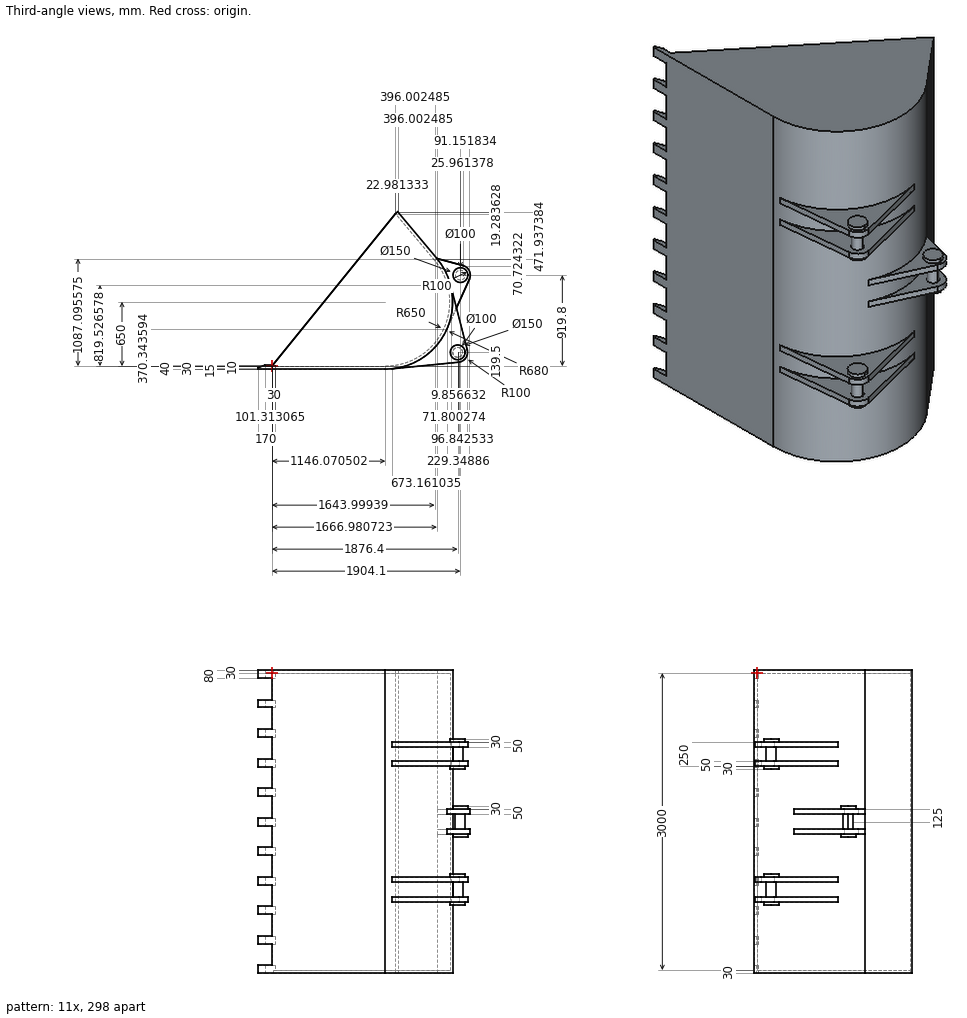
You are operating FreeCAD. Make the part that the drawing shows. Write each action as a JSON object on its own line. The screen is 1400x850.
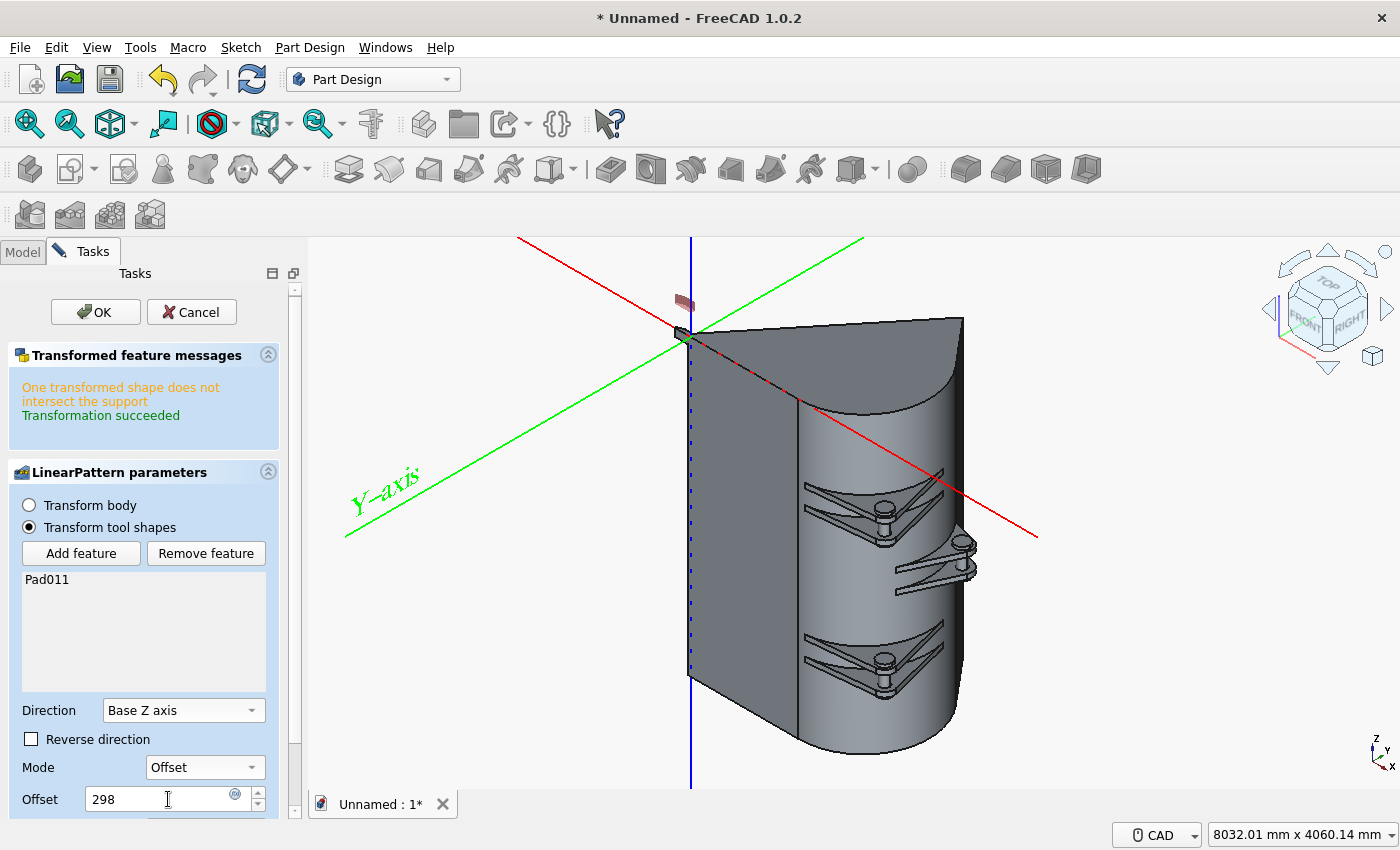
{"action": "scroll", "coordinate": [295, 550], "scroll_direction": "down", "scroll_amount": 2}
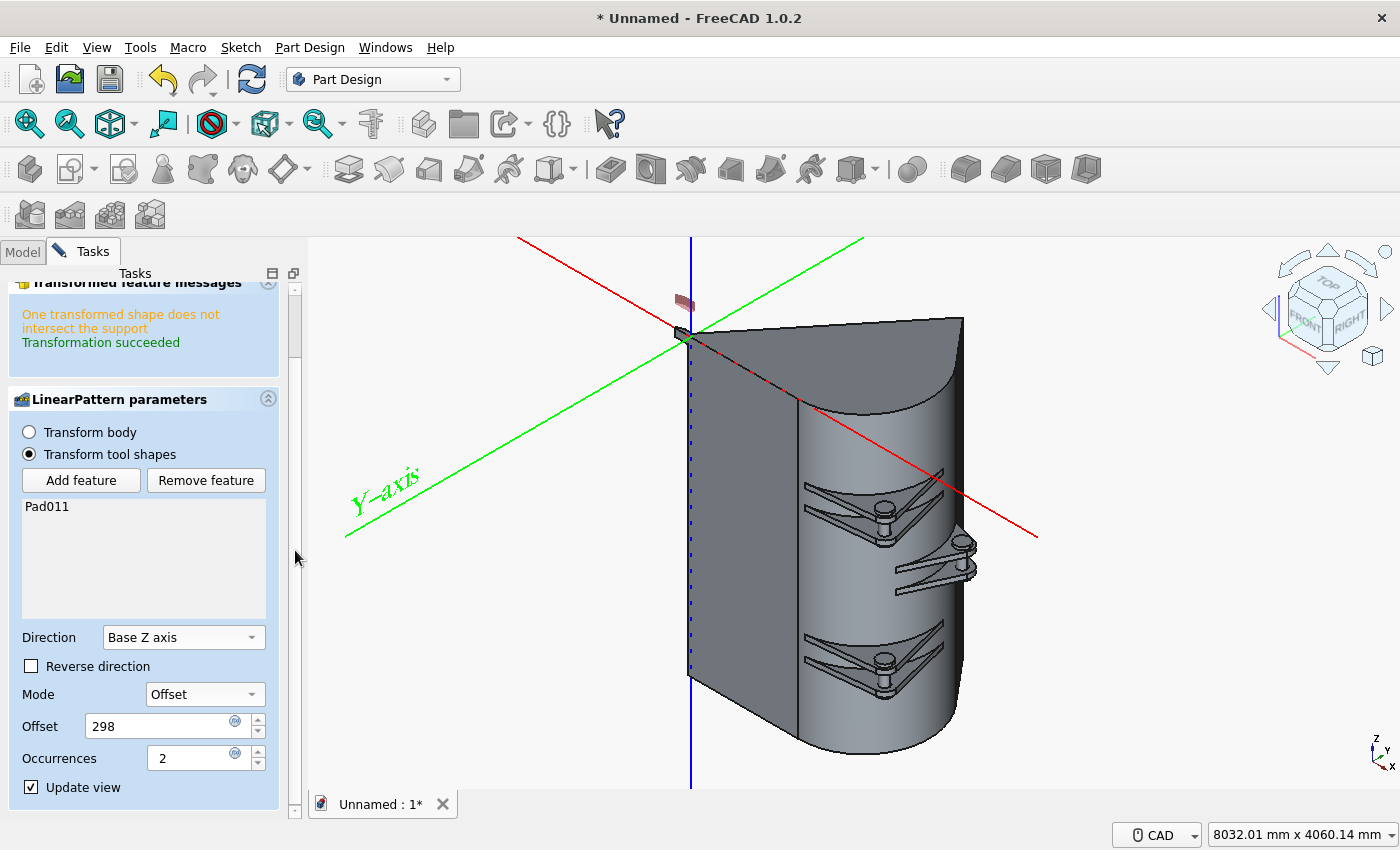
{"action": "triple_click", "coordinate": [198, 758]}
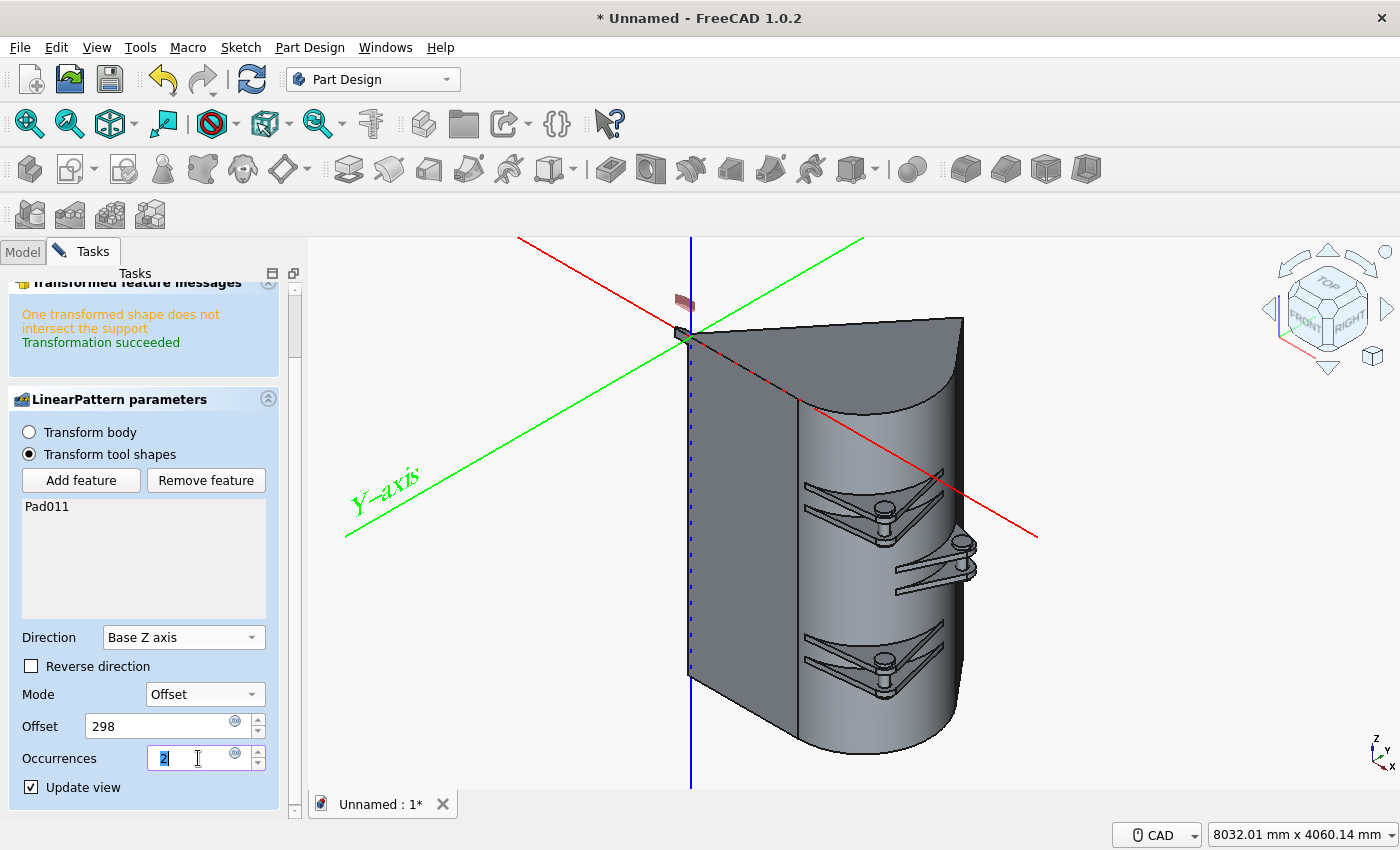
{"action": "type", "text": "11"}
{"action": "key", "text": "Tab"}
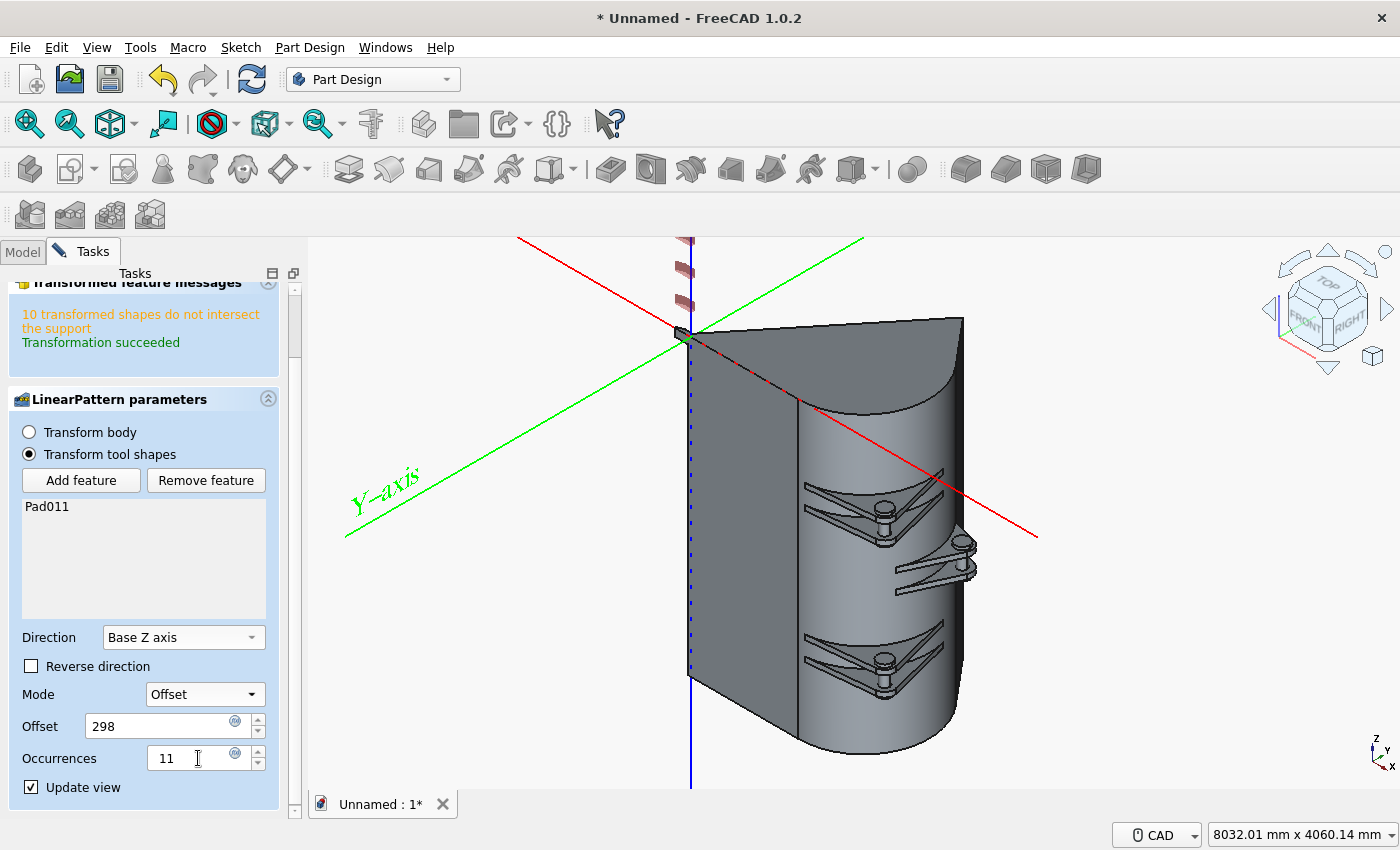
{"action": "left_click", "coordinate": [30, 666]}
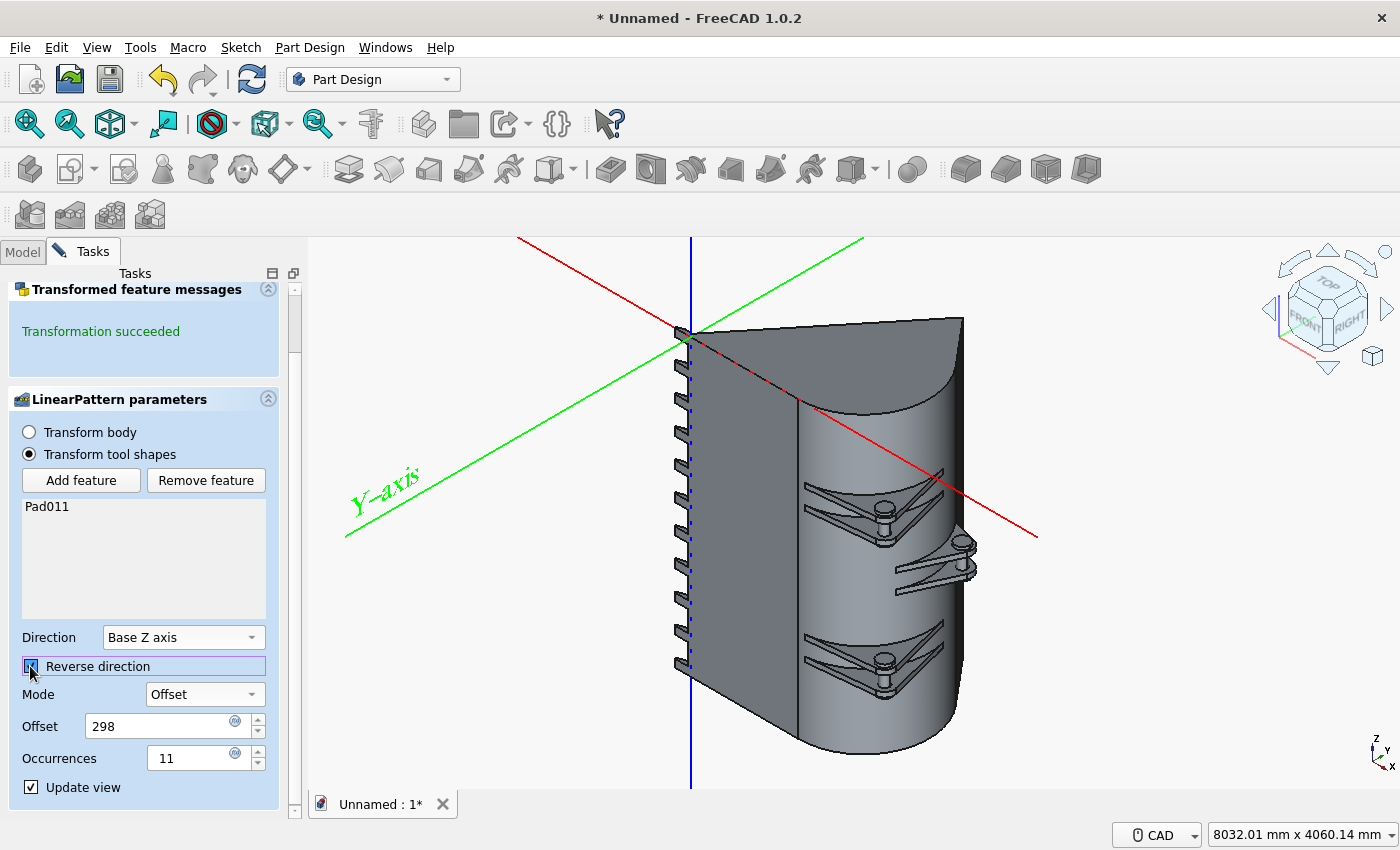
{"action": "scroll", "coordinate": [295, 550], "scroll_direction": "up", "scroll_amount": 2}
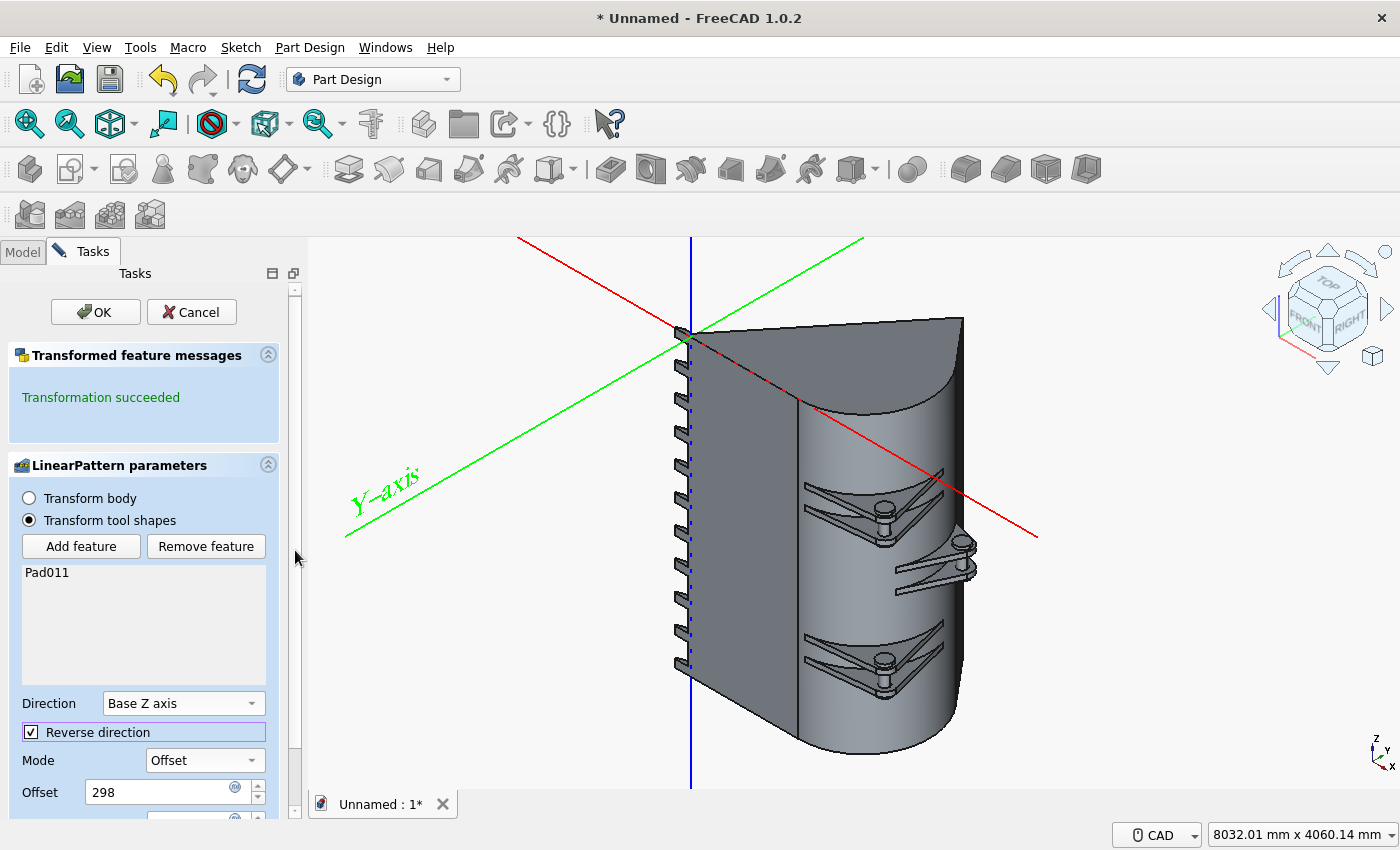
{"action": "left_click", "coordinate": [96, 312]}